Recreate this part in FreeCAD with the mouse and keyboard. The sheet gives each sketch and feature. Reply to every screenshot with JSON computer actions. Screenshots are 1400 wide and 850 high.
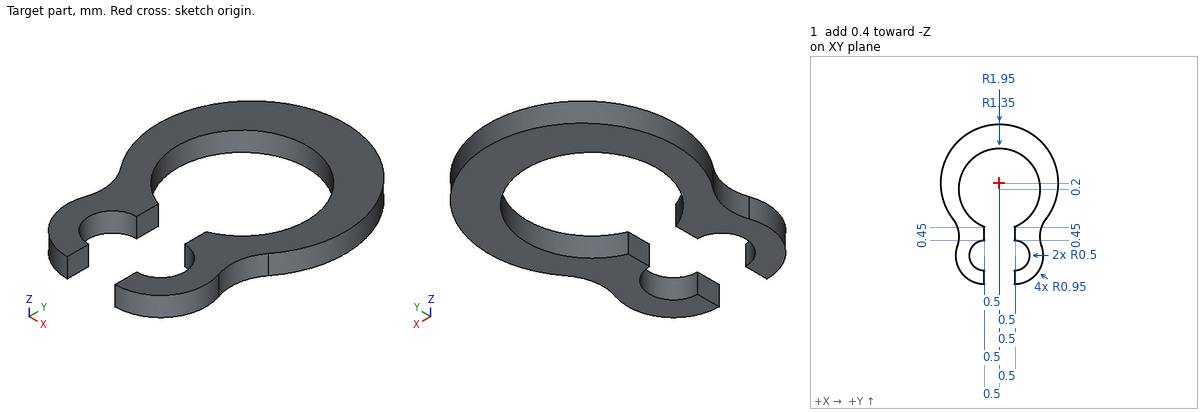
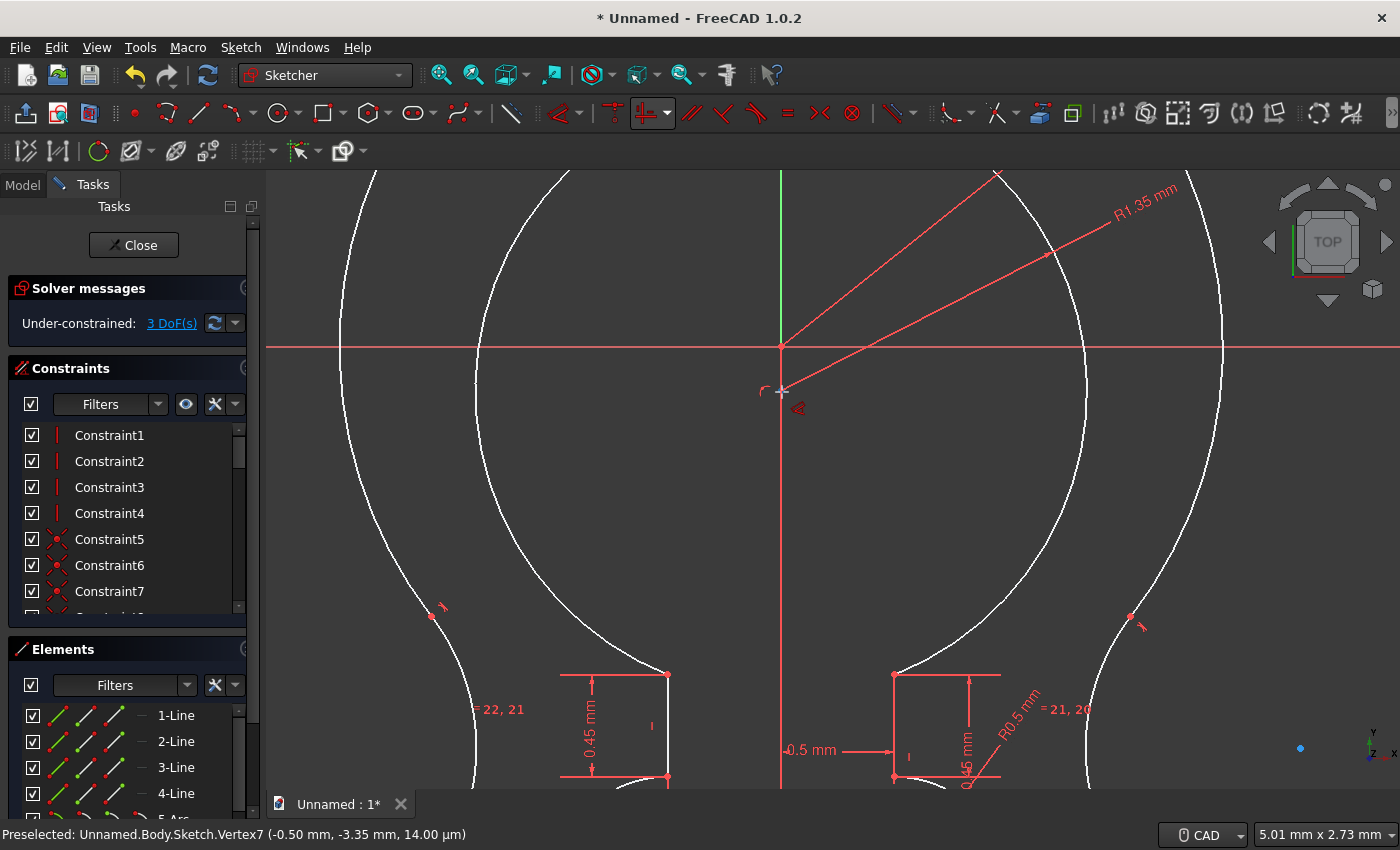
{"action": "left_click", "coordinate": [781, 391]}
{"action": "left_click", "coordinate": [815, 369]}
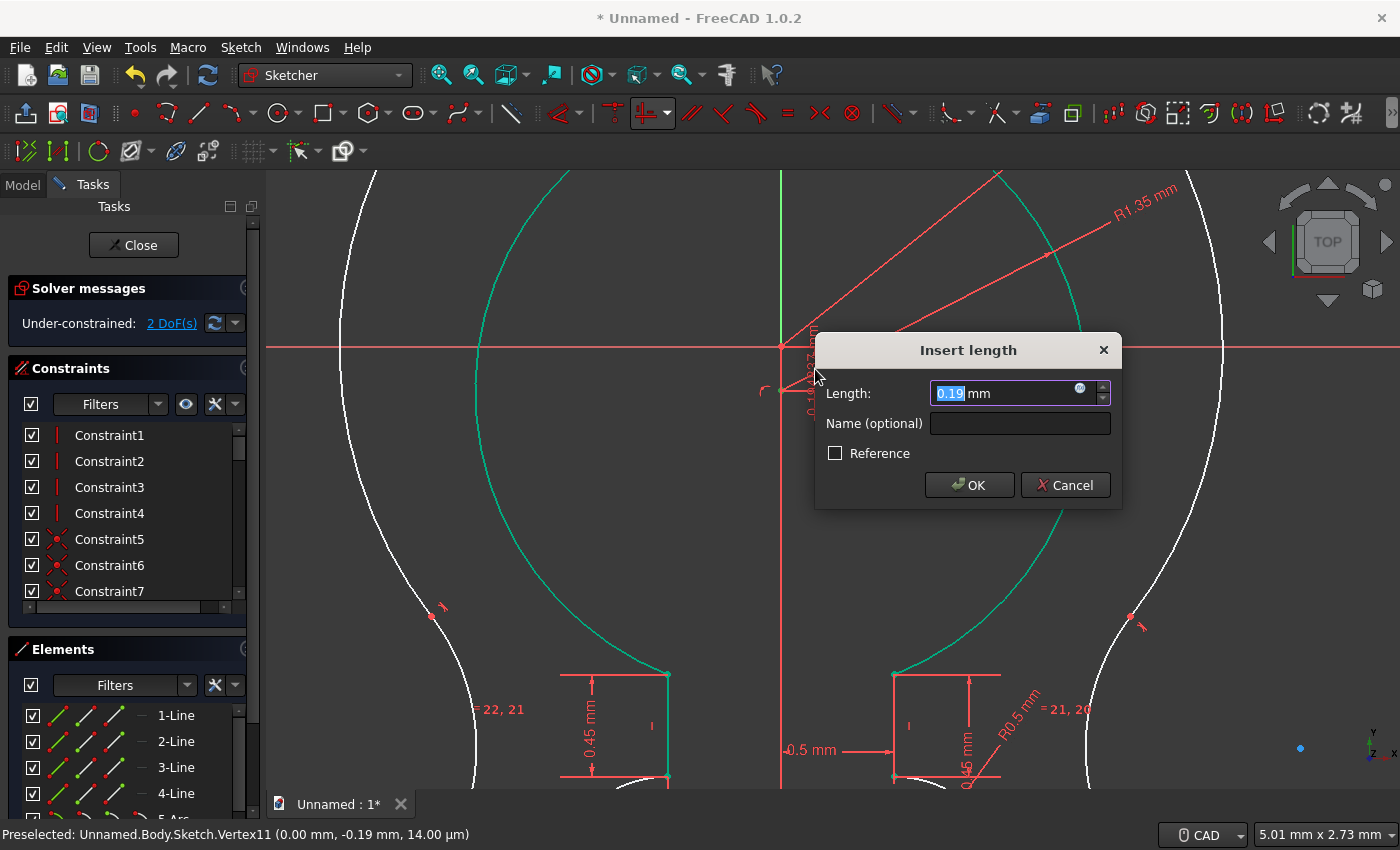
{"action": "type", "text": "0.2"}
{"action": "key", "text": "Return"}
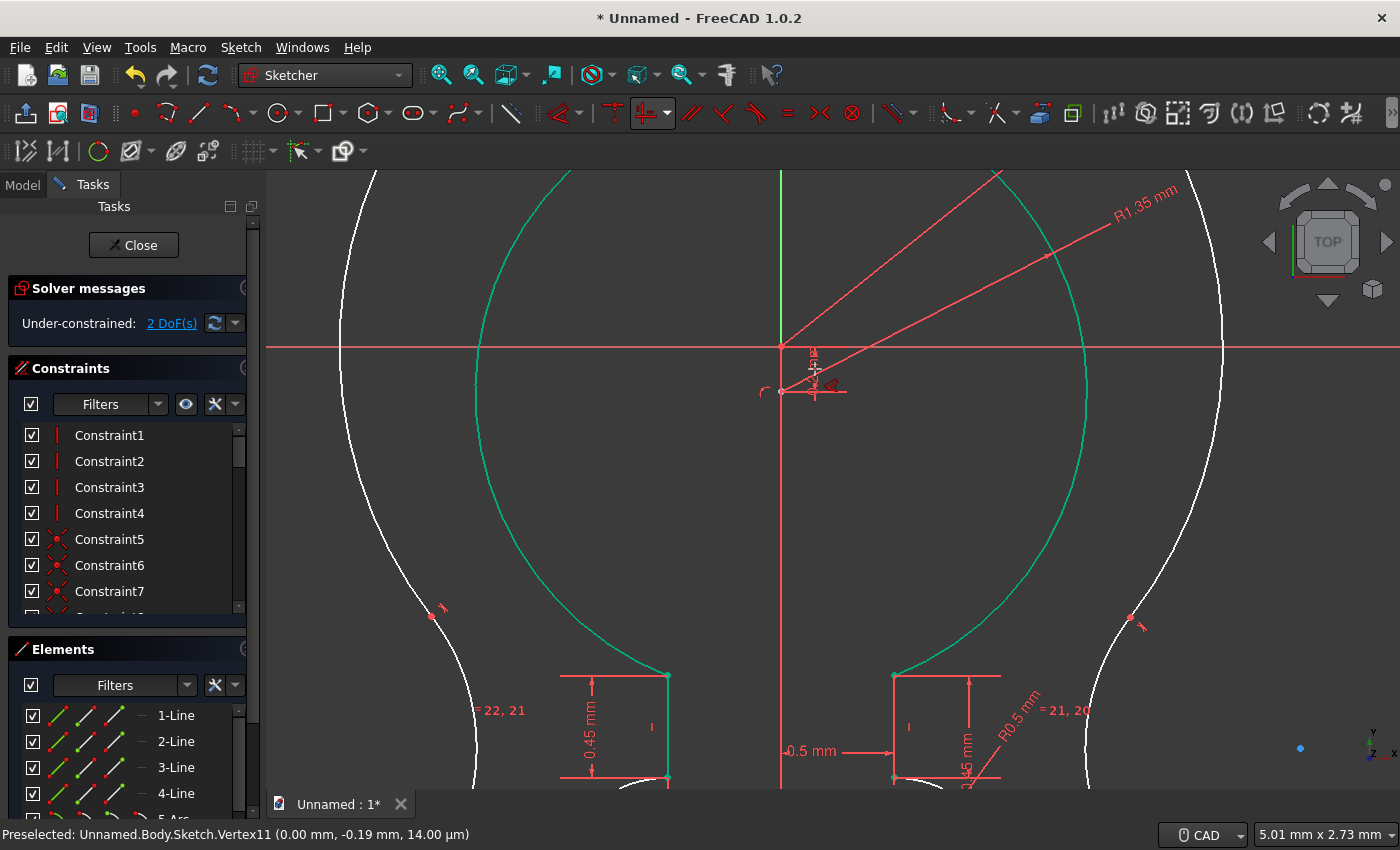
{"action": "scroll", "coordinate": [757, 468], "scroll_direction": "down", "scroll_amount": 6}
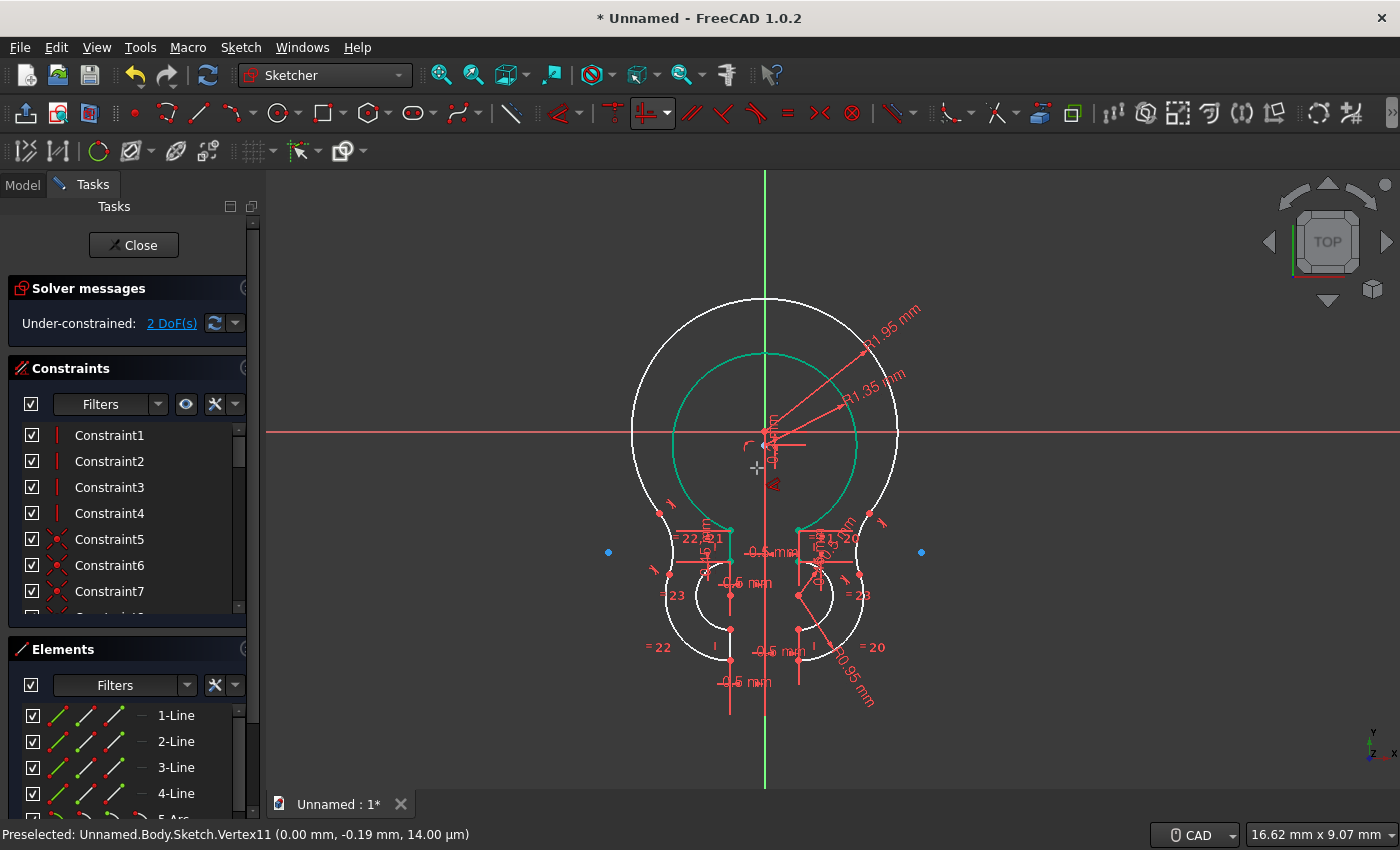
{"action": "left_click", "coordinate": [799, 596]}
{"action": "left_click", "coordinate": [782, 630]}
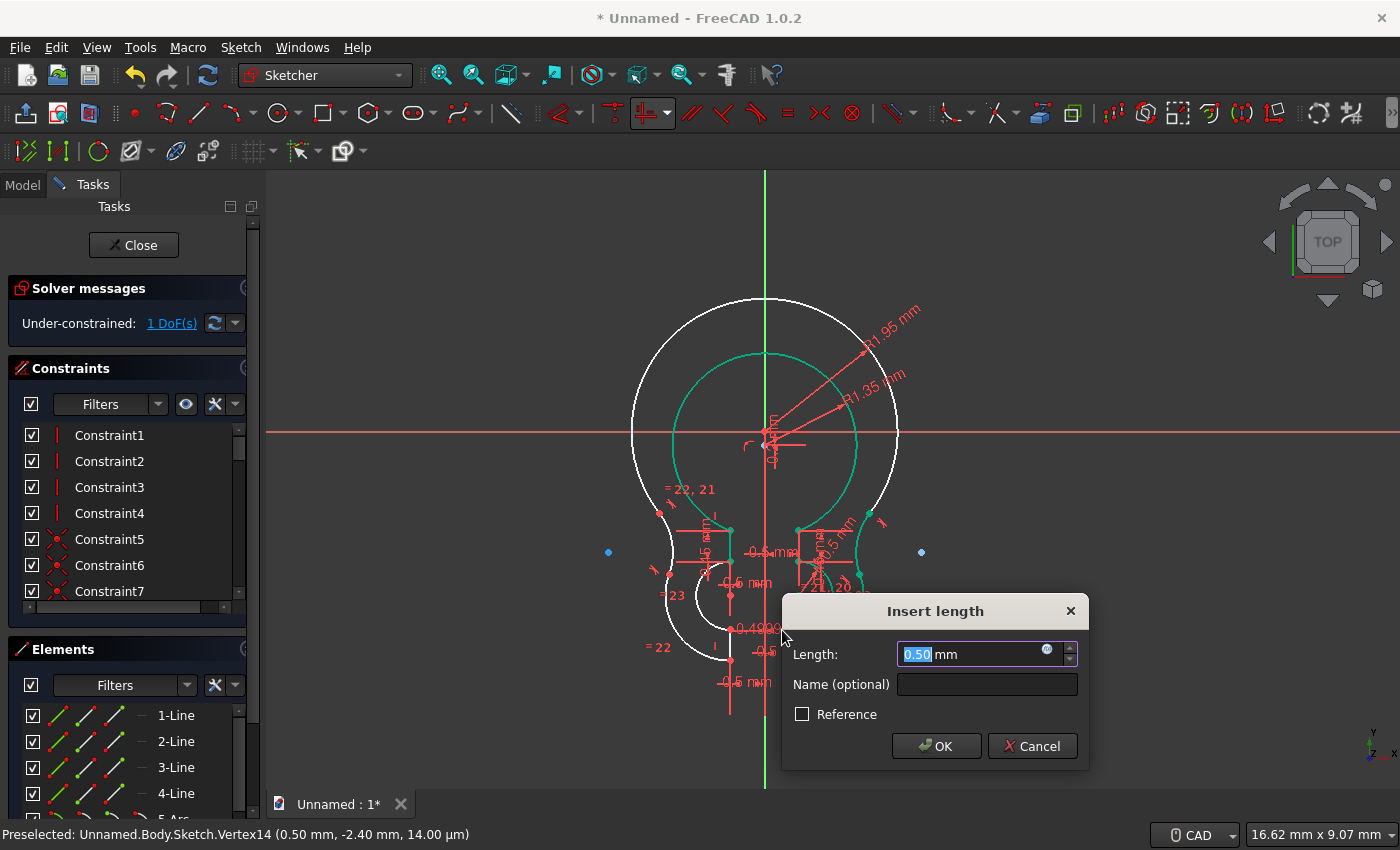
{"action": "type", "text": "0.5"}
{"action": "key", "text": "Return"}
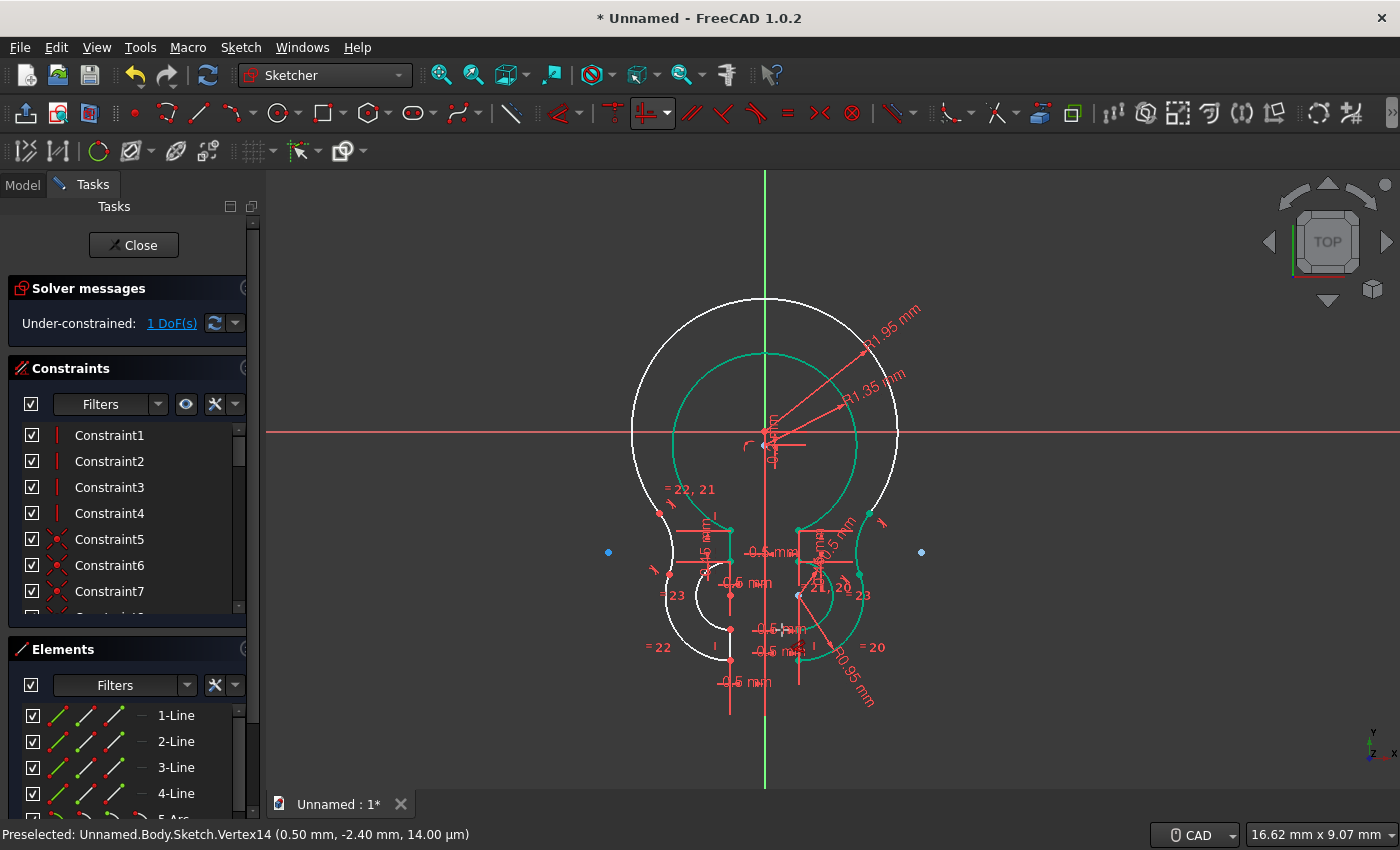
{"action": "left_click", "coordinate": [730, 596]}
{"action": "left_click", "coordinate": [747, 398]}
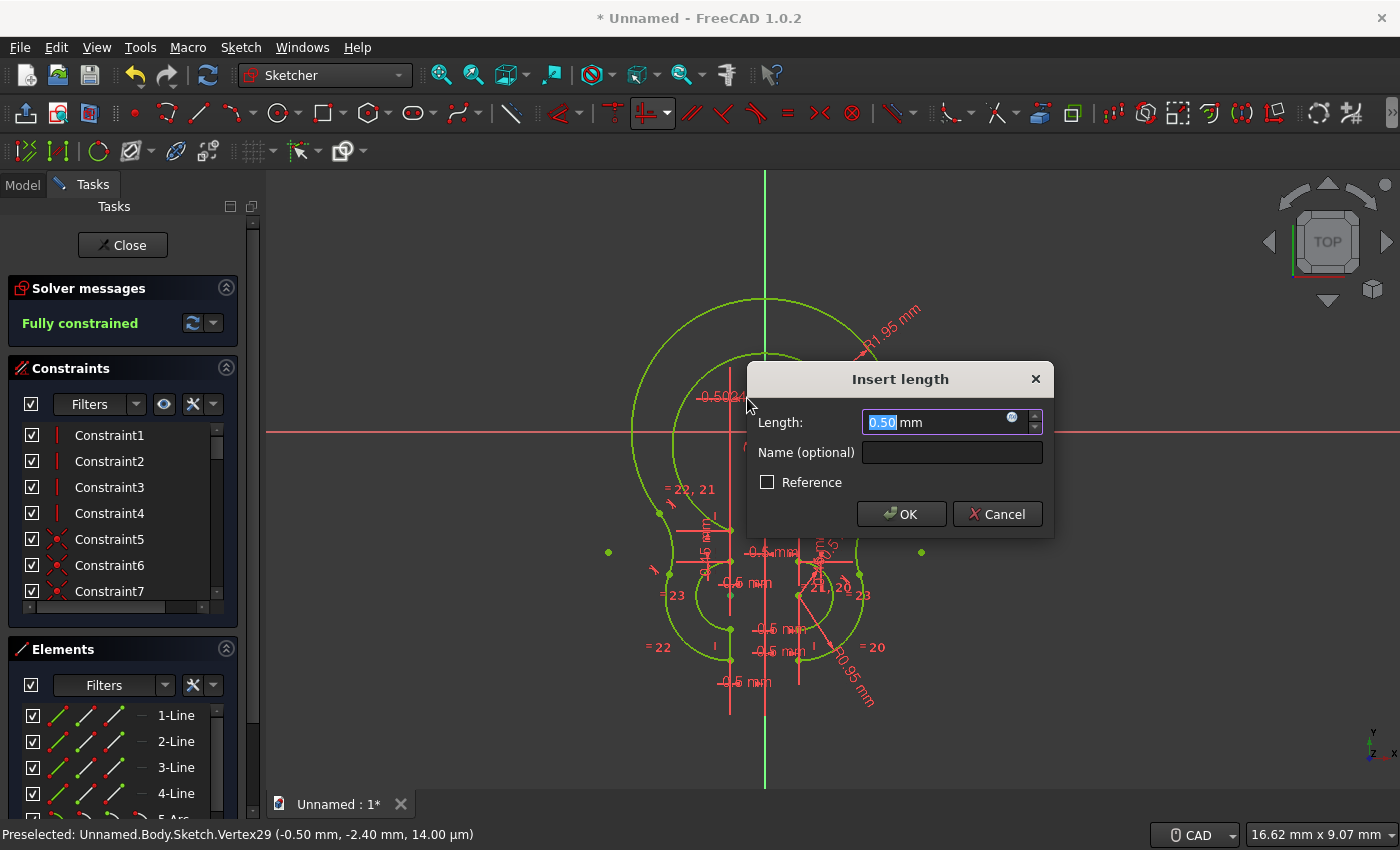
{"action": "type", "text": "0.5"}
{"action": "key", "text": "Return"}
{"action": "key", "text": "Escape"}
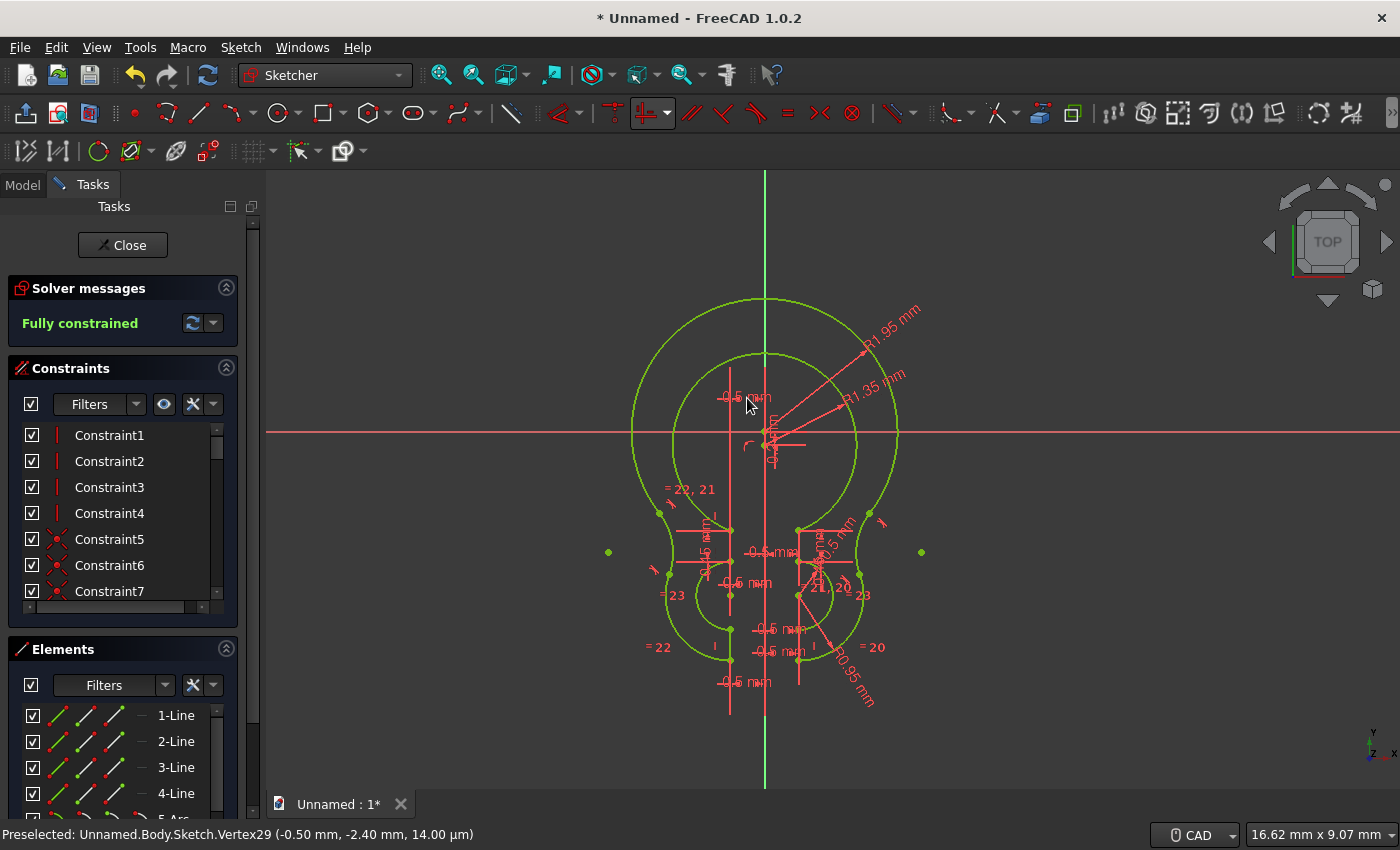
{"action": "left_click", "coordinate": [123, 245]}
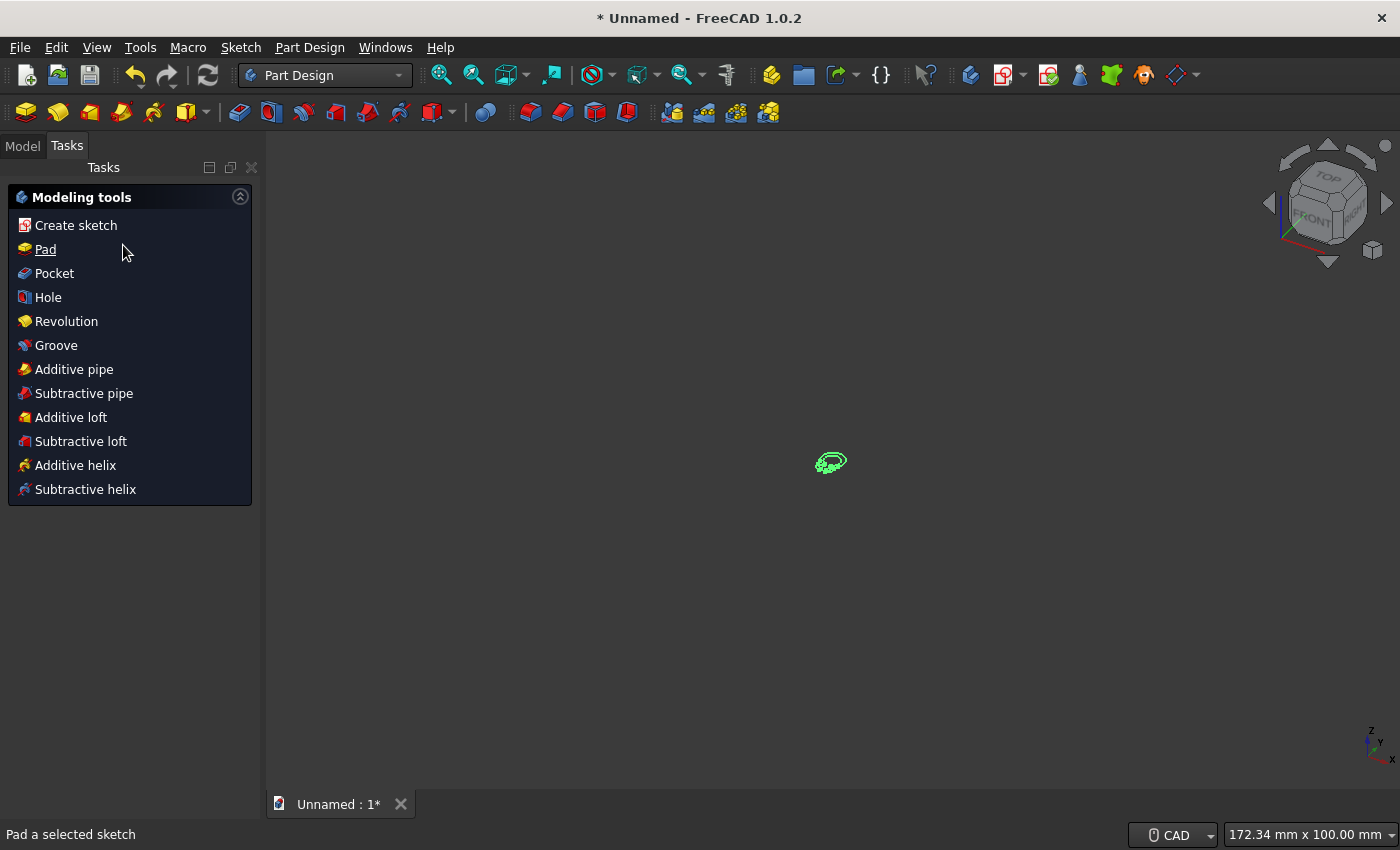
{"action": "left_click", "coordinate": [26, 112]}